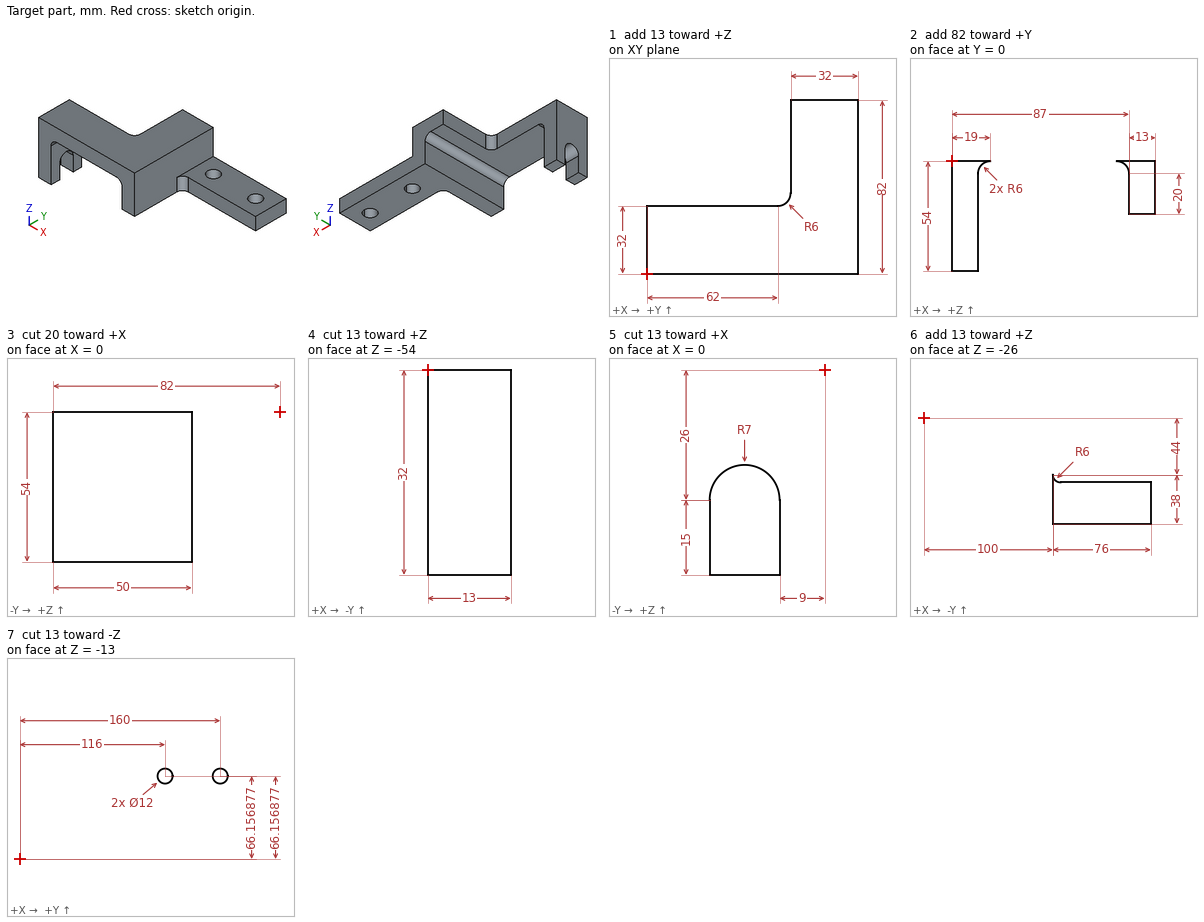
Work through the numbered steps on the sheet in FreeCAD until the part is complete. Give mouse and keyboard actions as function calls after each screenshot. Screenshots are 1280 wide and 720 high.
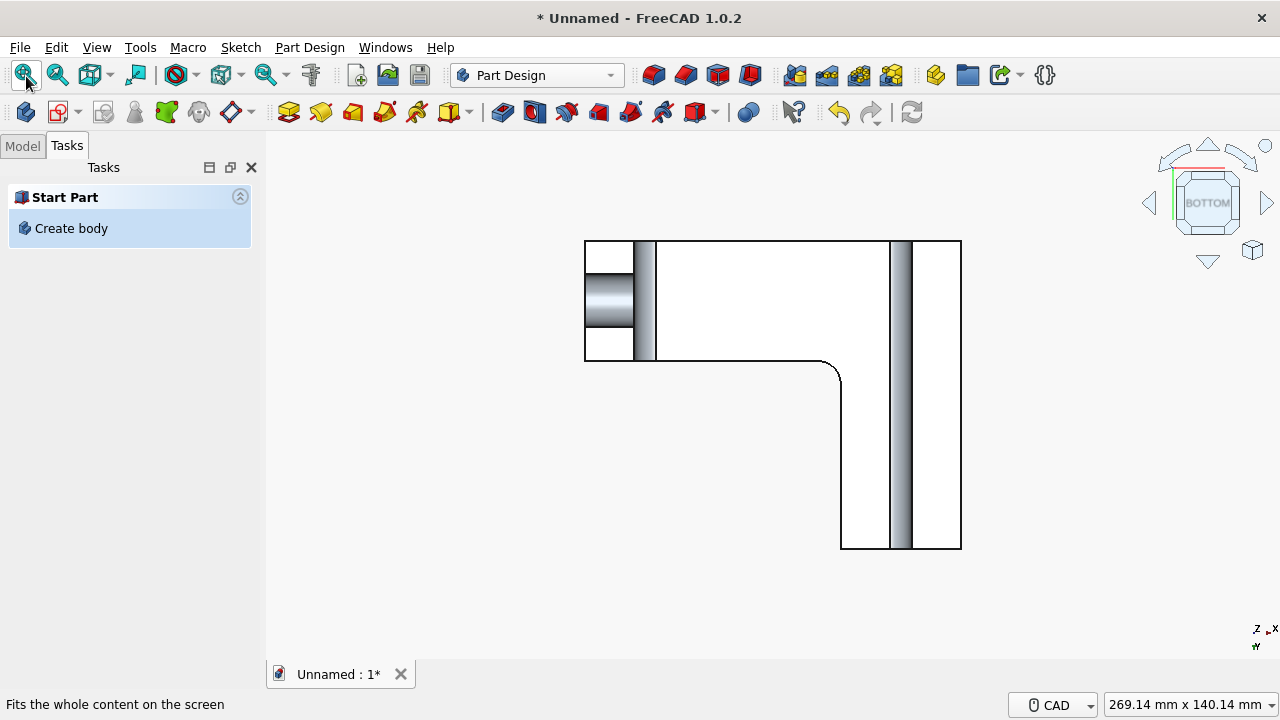
click(937, 482)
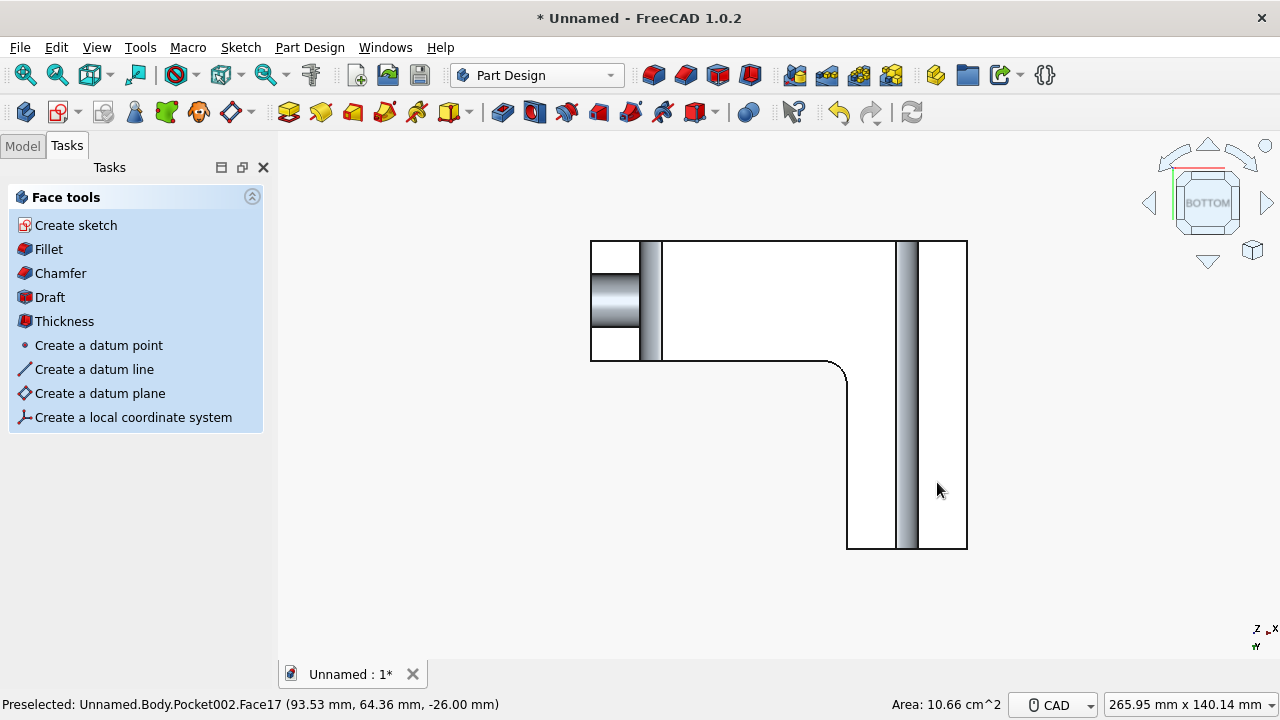
click(58, 112)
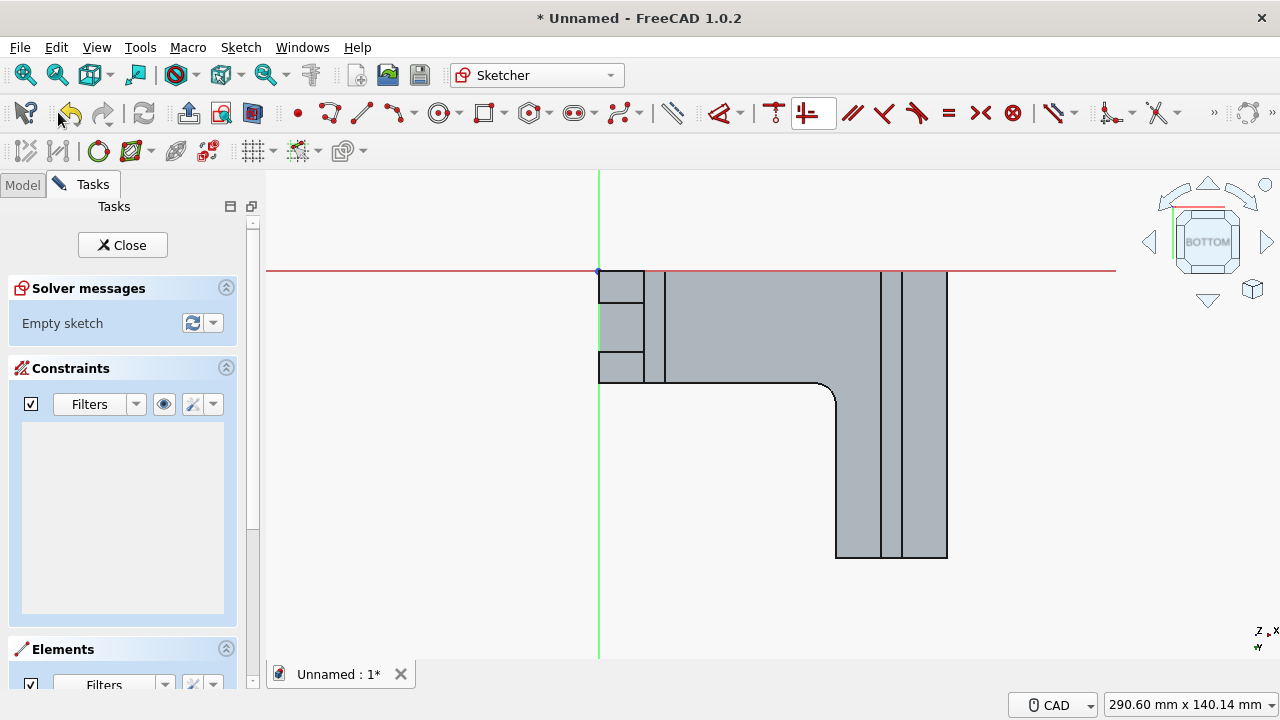
scroll(294, 415, down, 1)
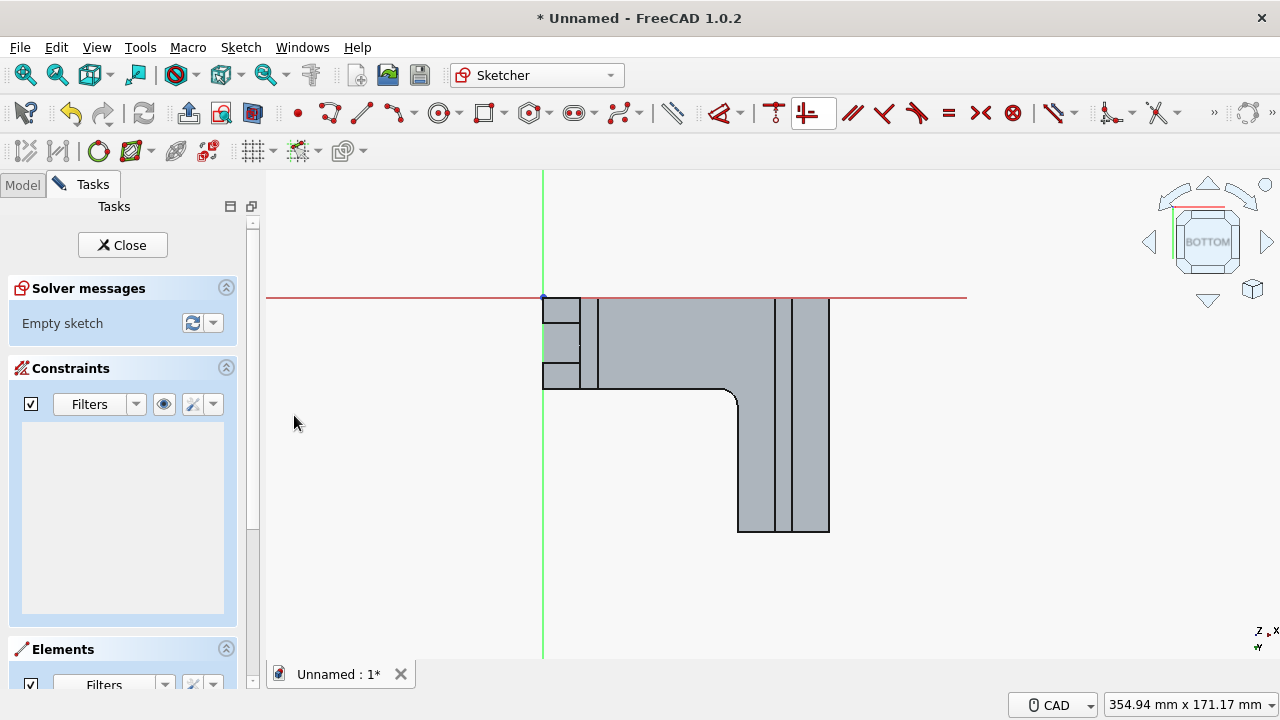
click(330, 114)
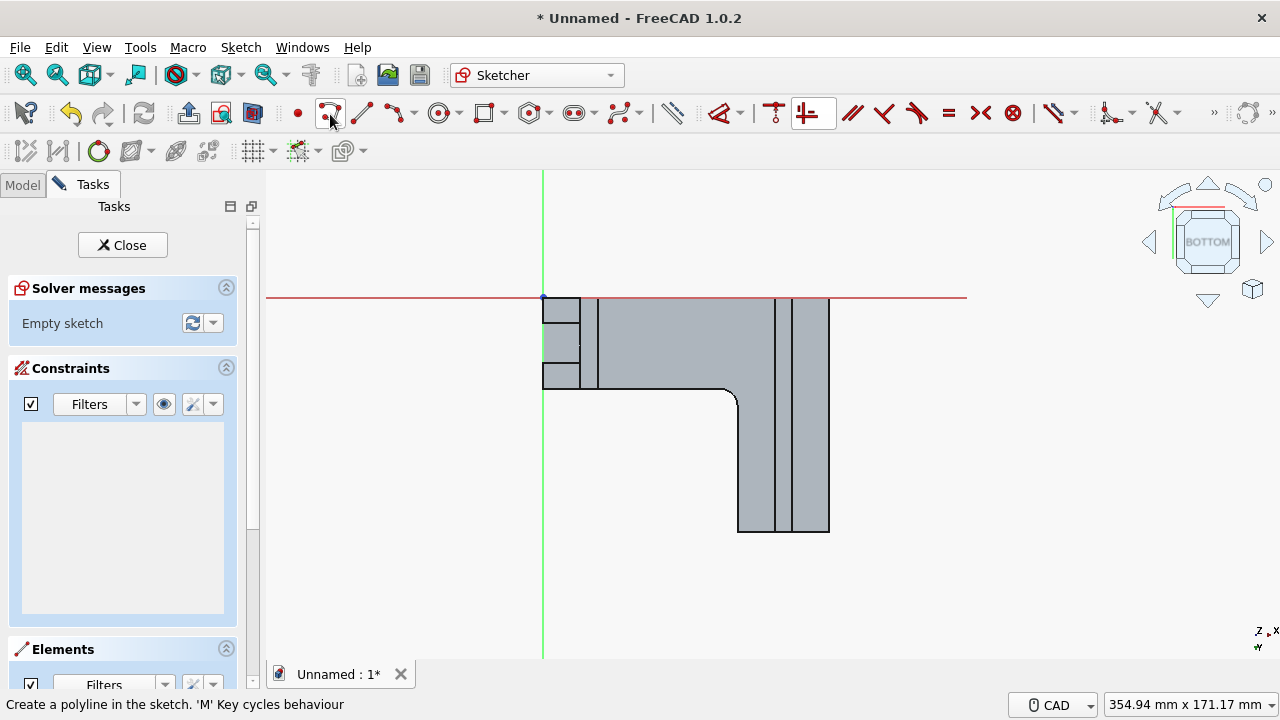
click(829, 423)
click(829, 532)
click(1046, 532)
click(1046, 440)
click(846, 440)
right_click(846, 440)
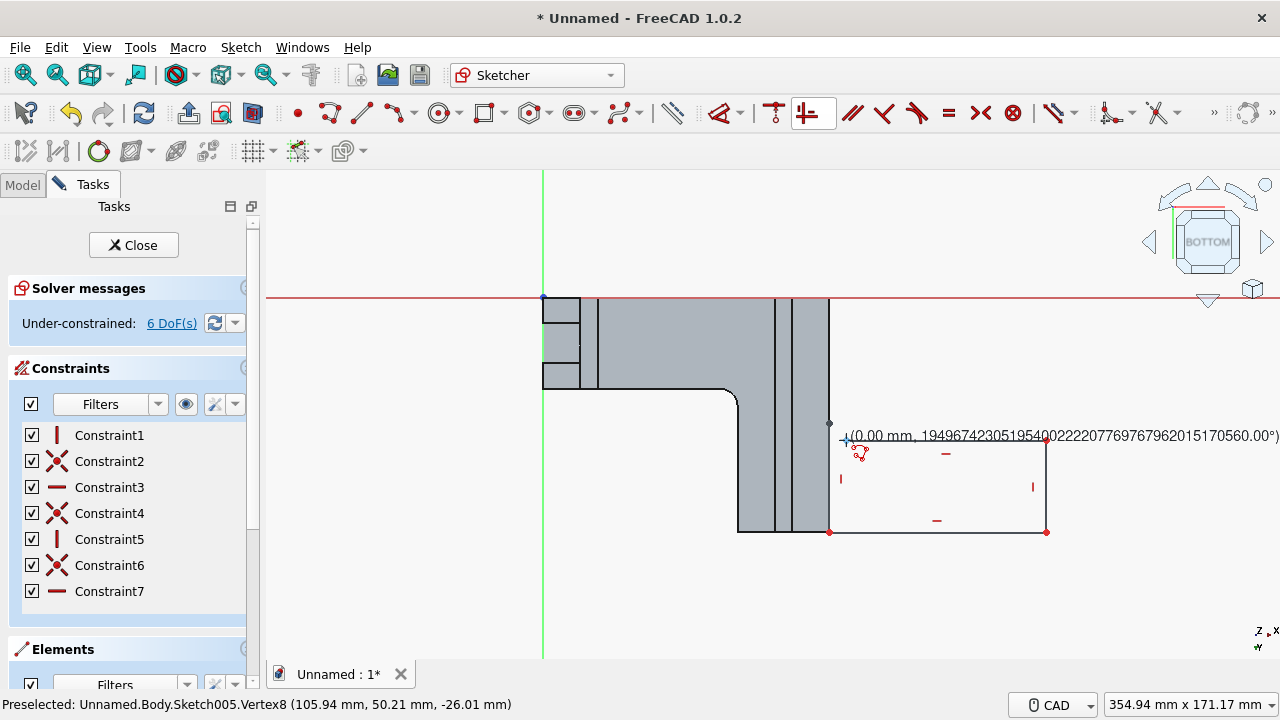
click(394, 114)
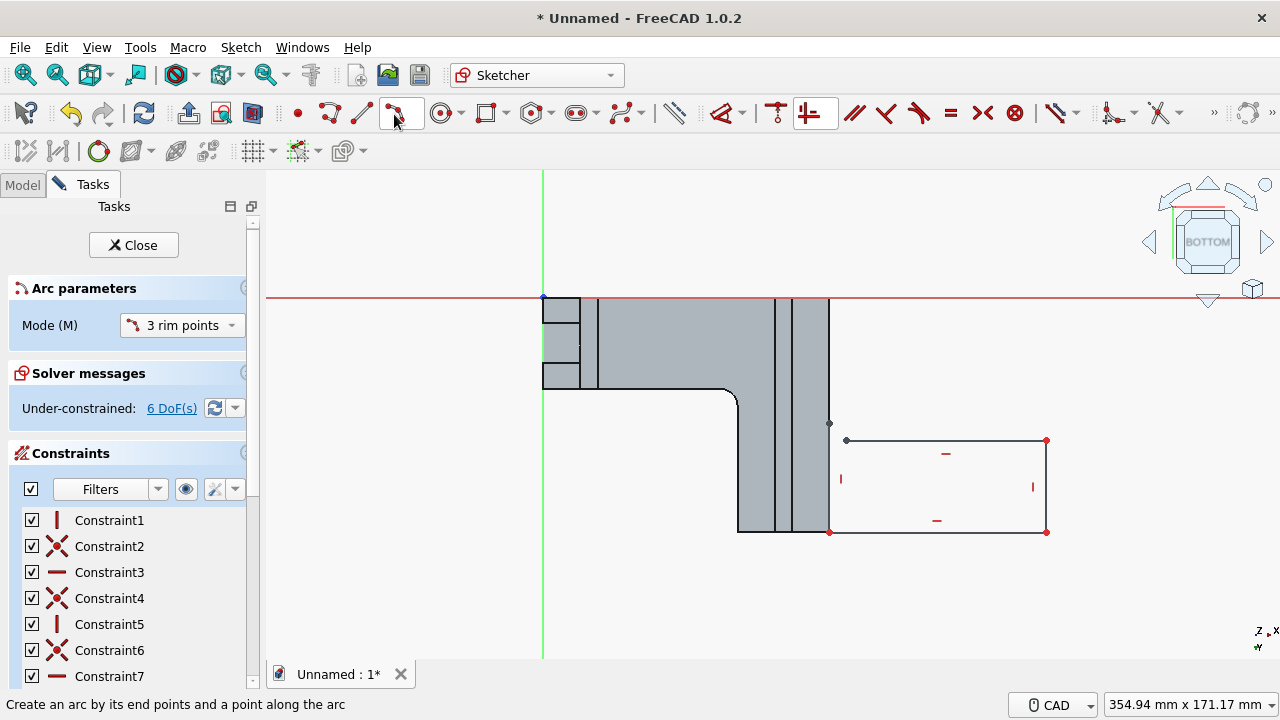
click(846, 441)
click(829, 424)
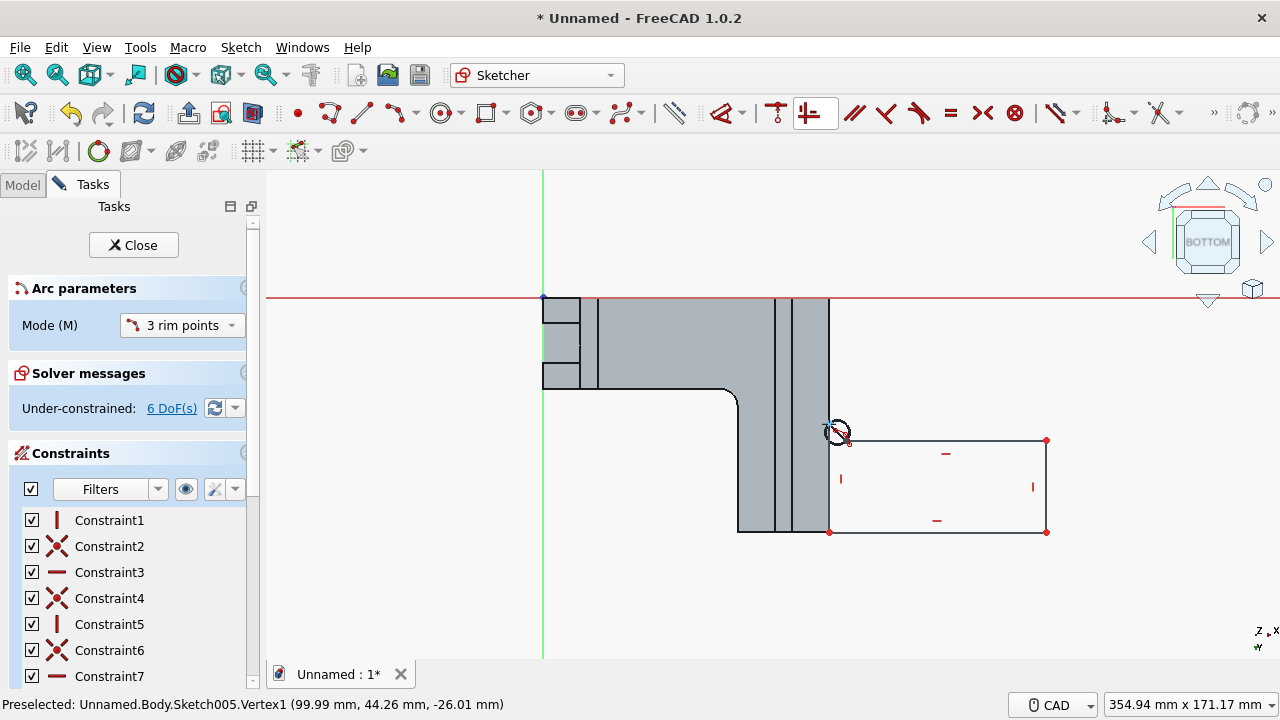
scroll(834, 435, up, 6)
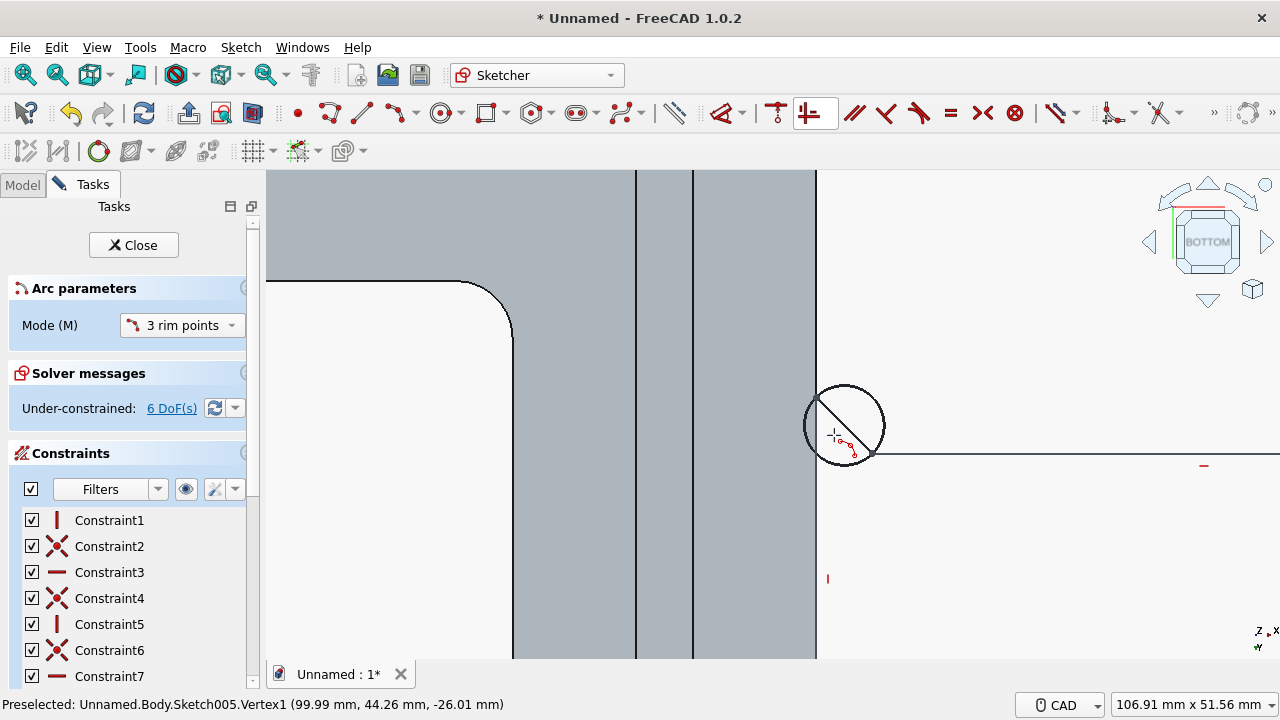
click(833, 435)
key(Escape)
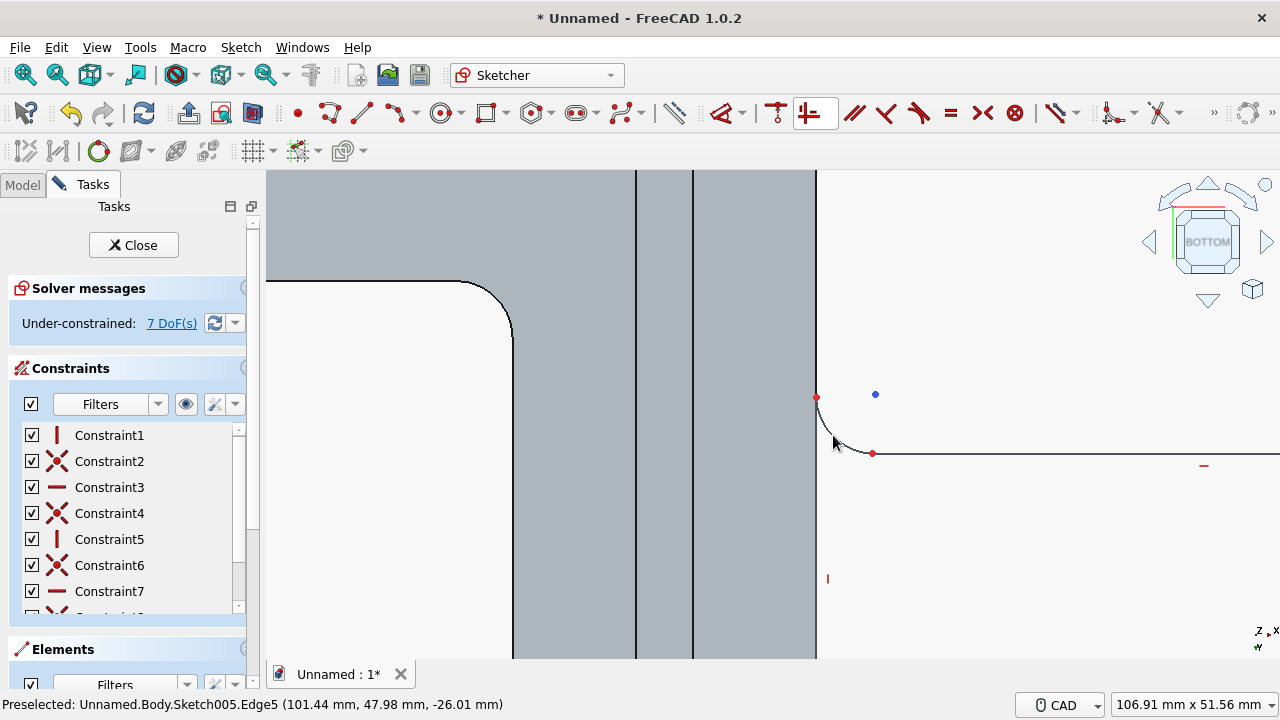
click(816, 506)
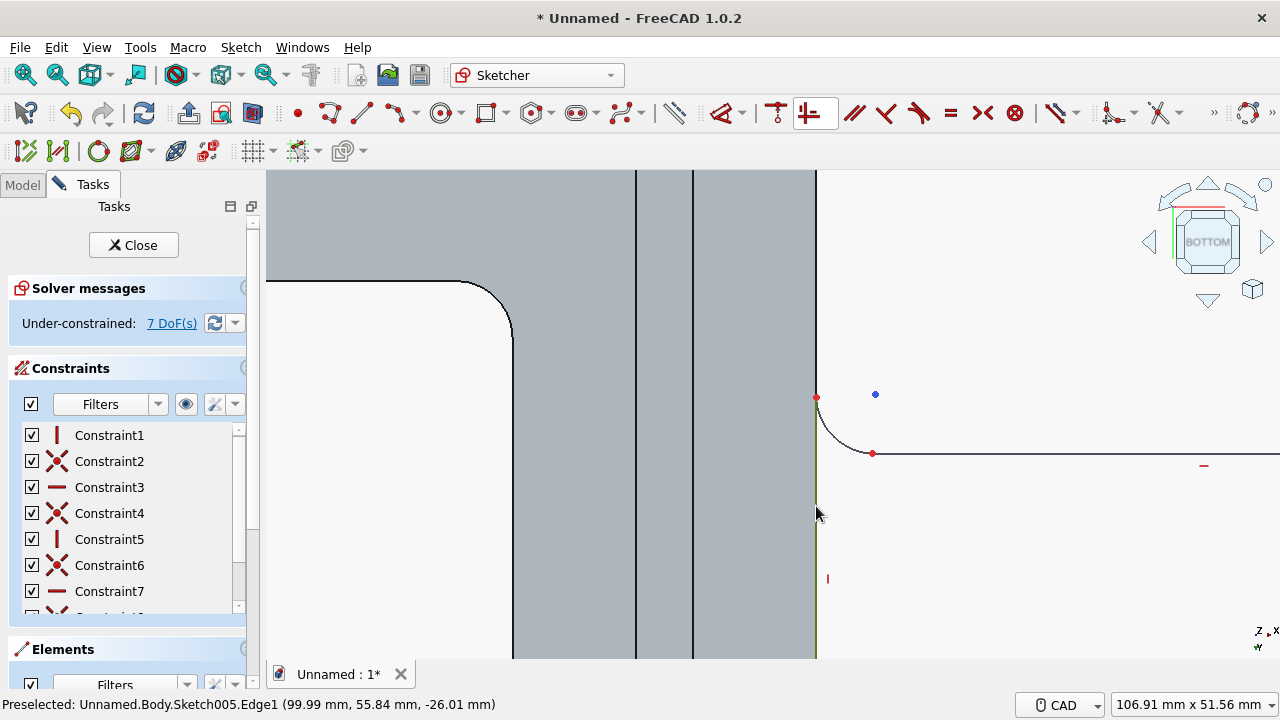
click(847, 447)